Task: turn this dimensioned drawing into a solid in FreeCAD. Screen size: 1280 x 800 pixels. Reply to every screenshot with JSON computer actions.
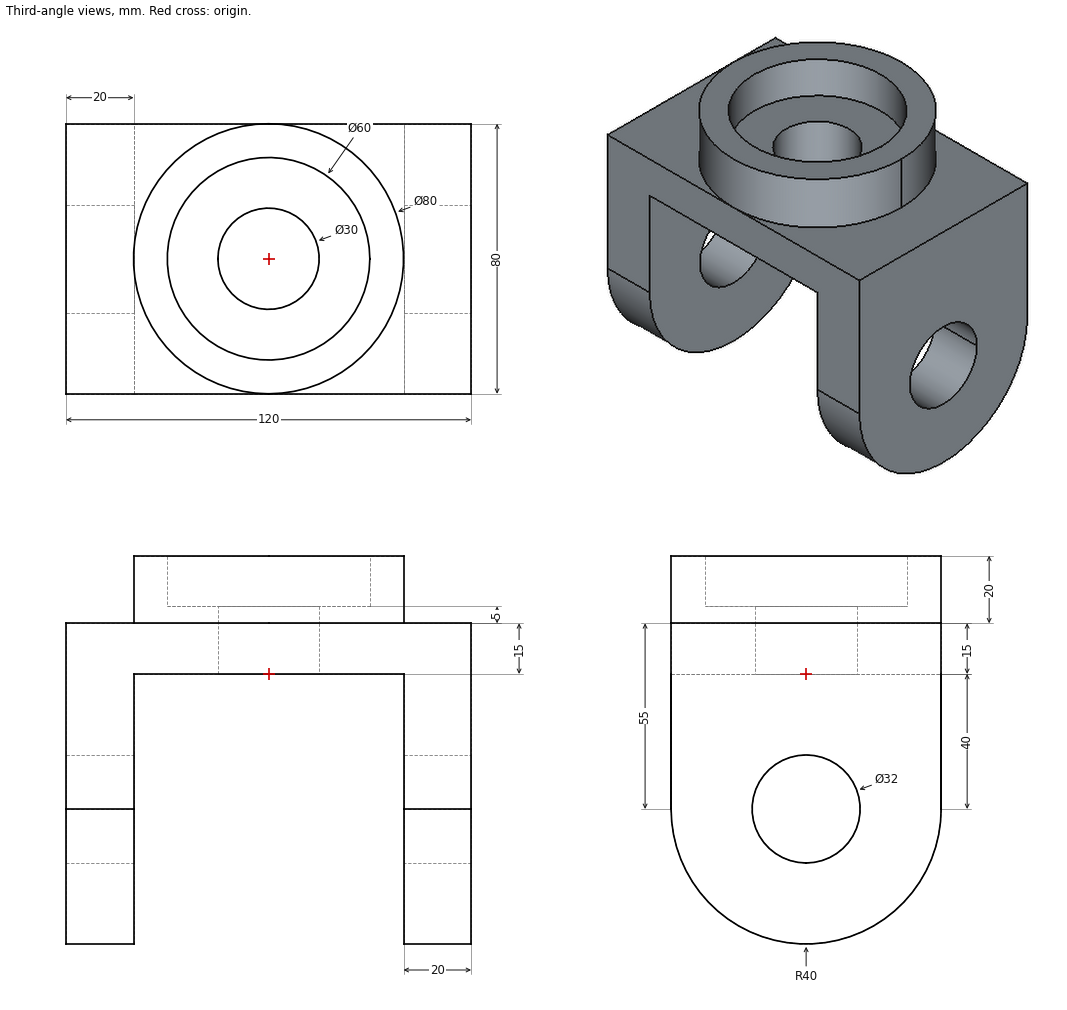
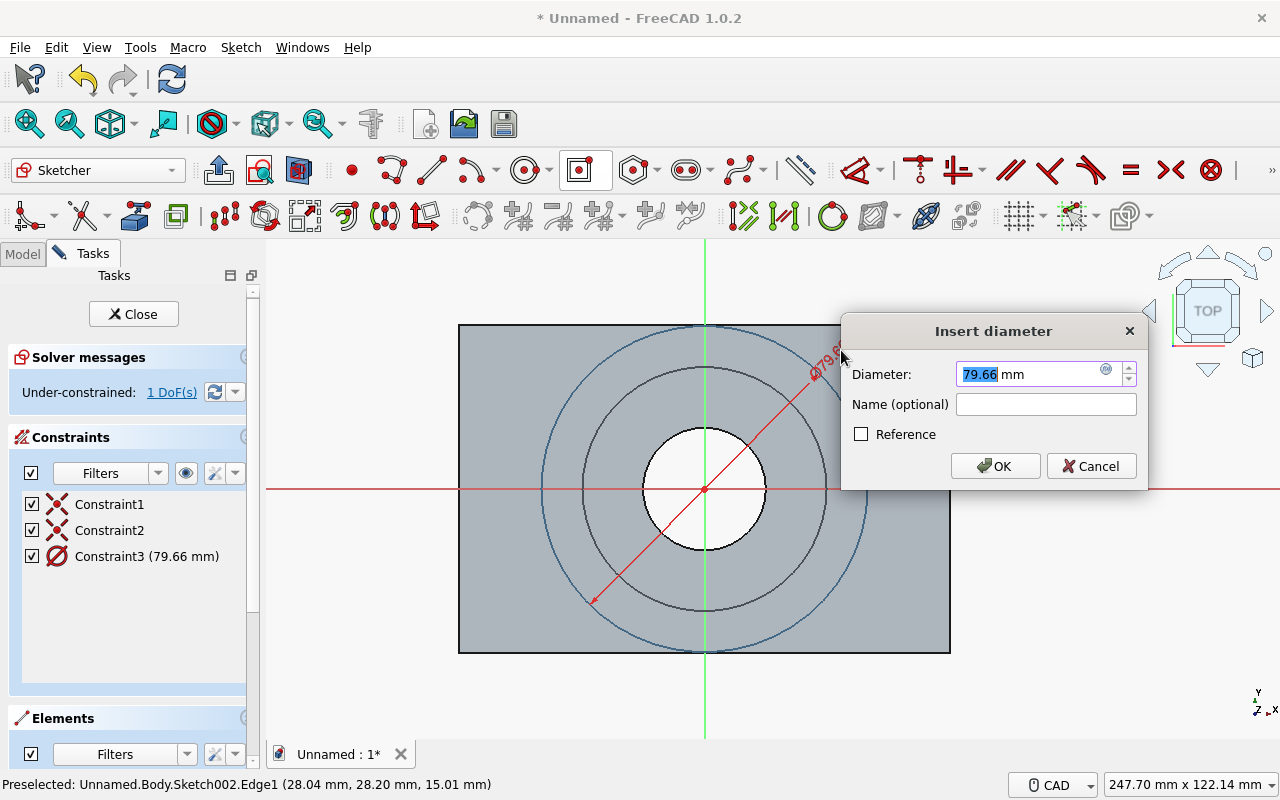
{"action": "type", "text": "80"}
{"action": "key", "text": "Return"}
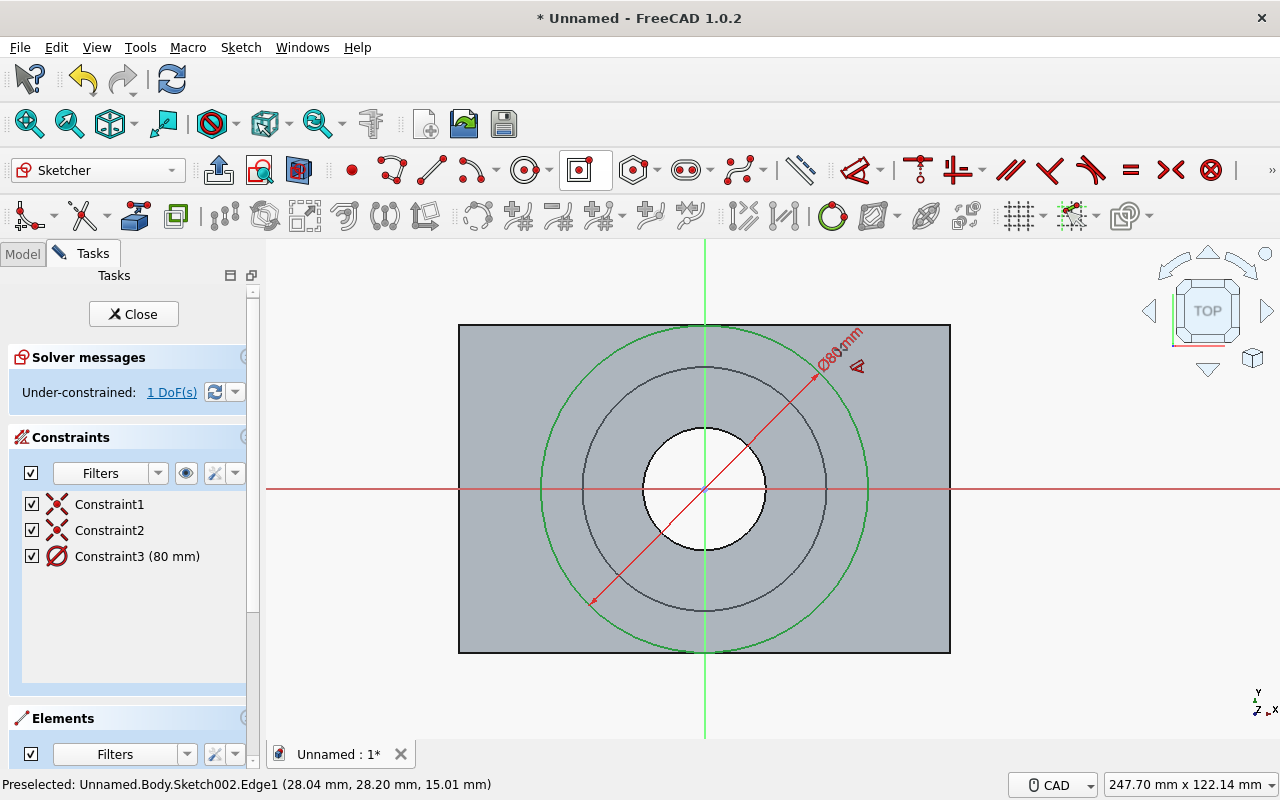
{"action": "left_click", "coordinate": [791, 403]}
{"action": "left_click", "coordinate": [874, 440]}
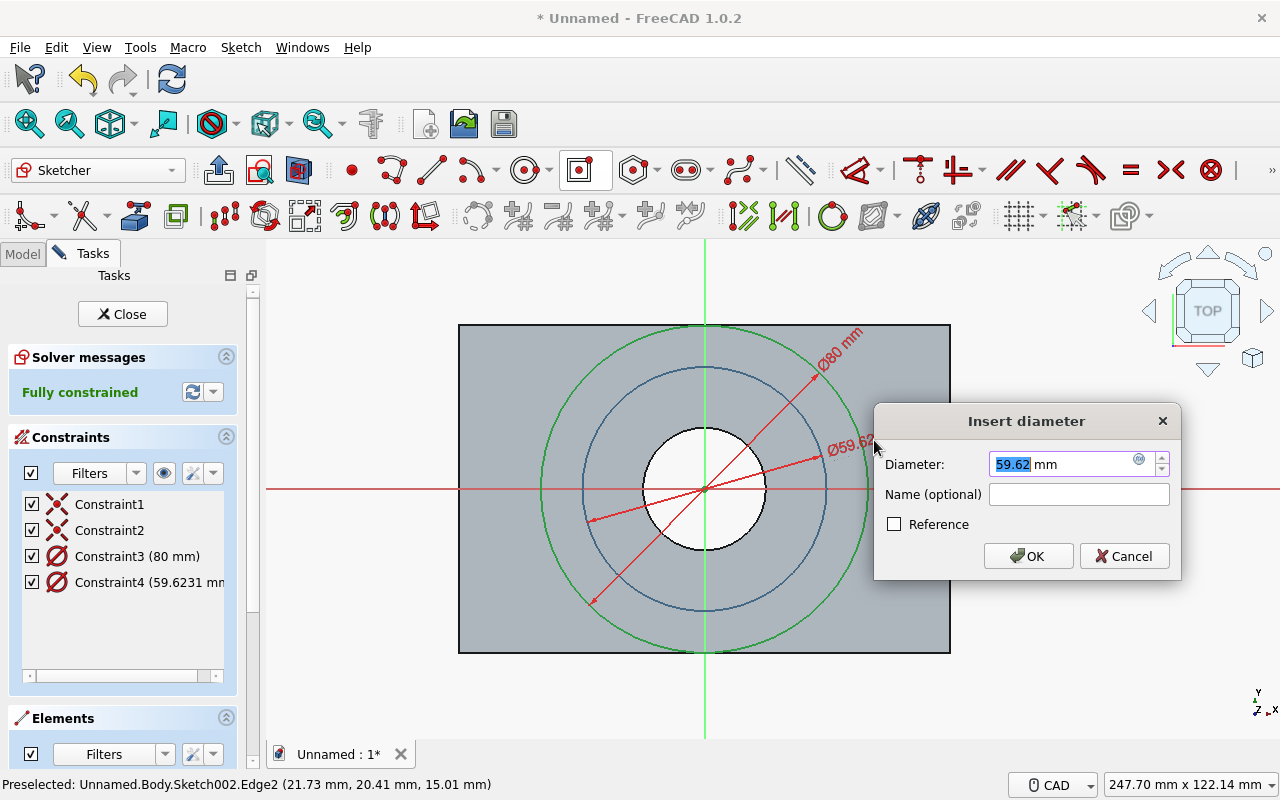
{"action": "type", "text": "60"}
{"action": "key", "text": "Return"}
{"action": "key", "text": "Escape"}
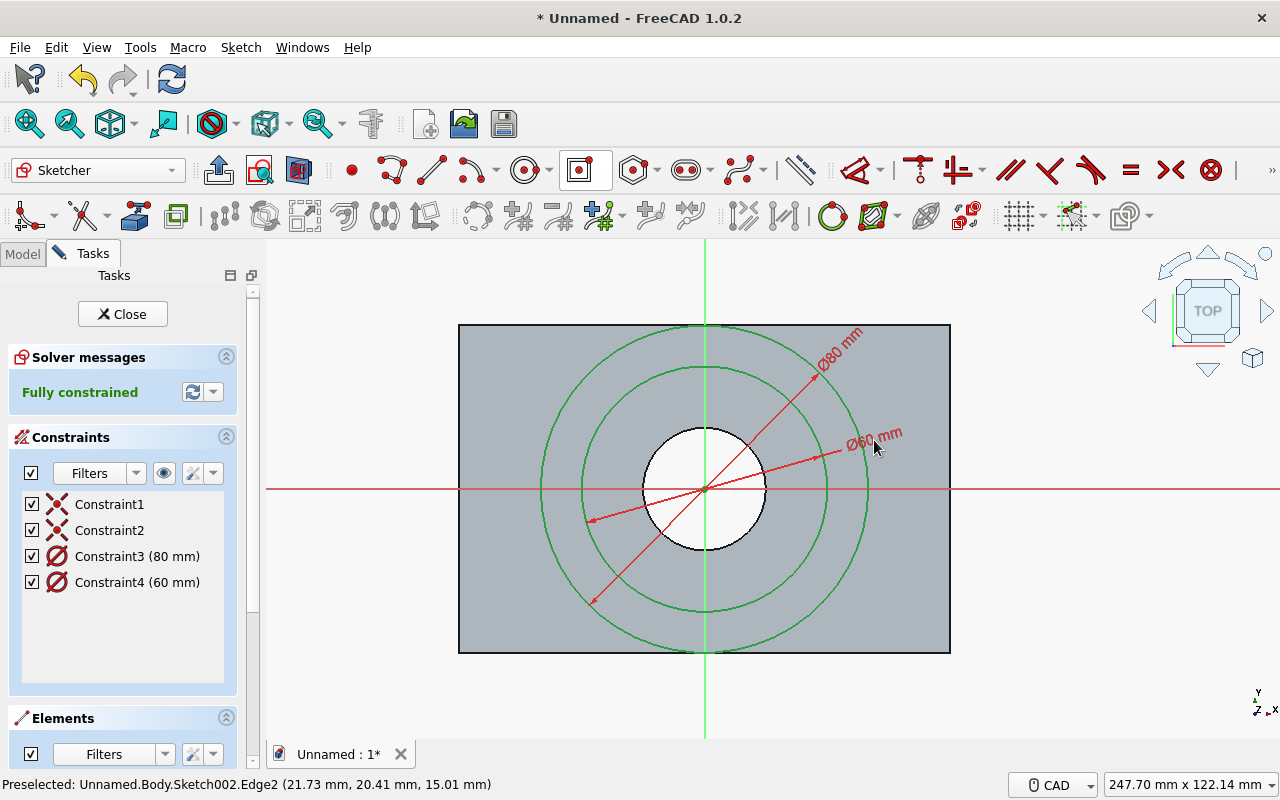
{"action": "left_click", "coordinate": [123, 314]}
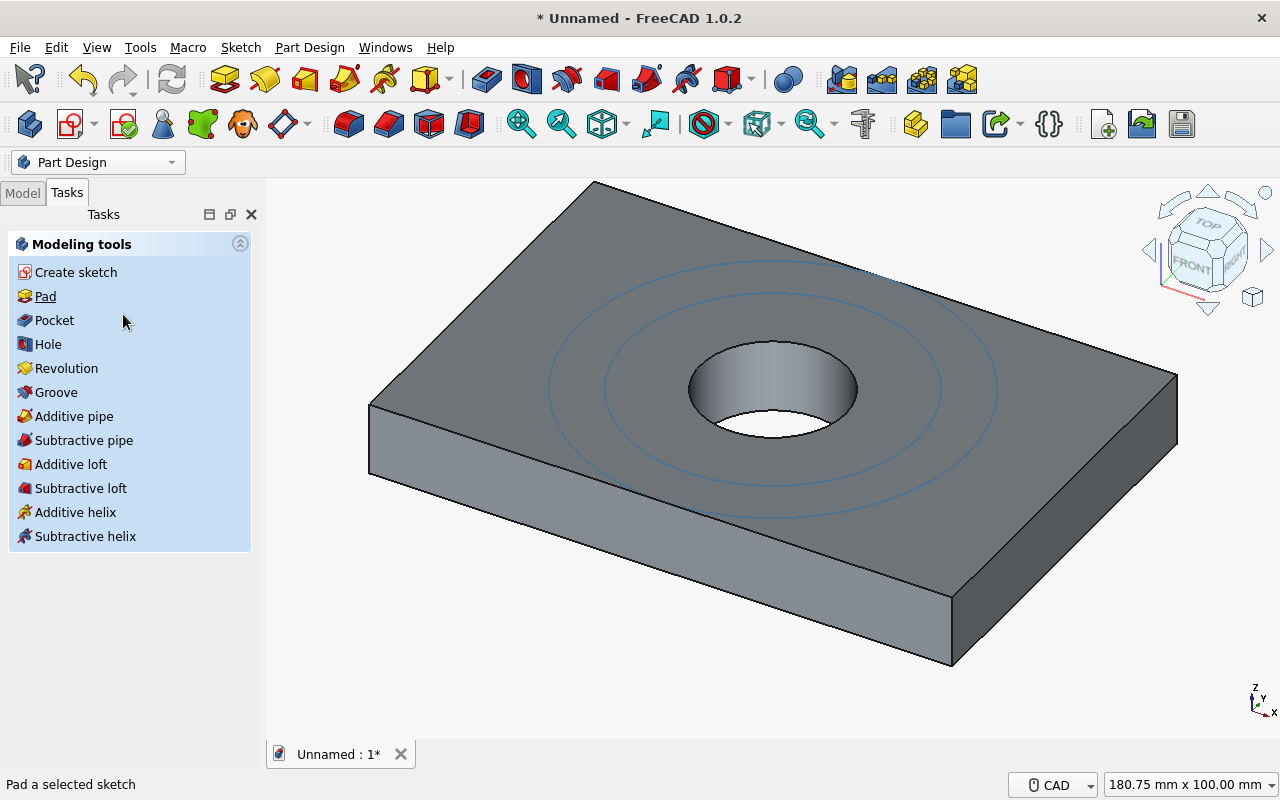
{"action": "left_click", "coordinate": [226, 80]}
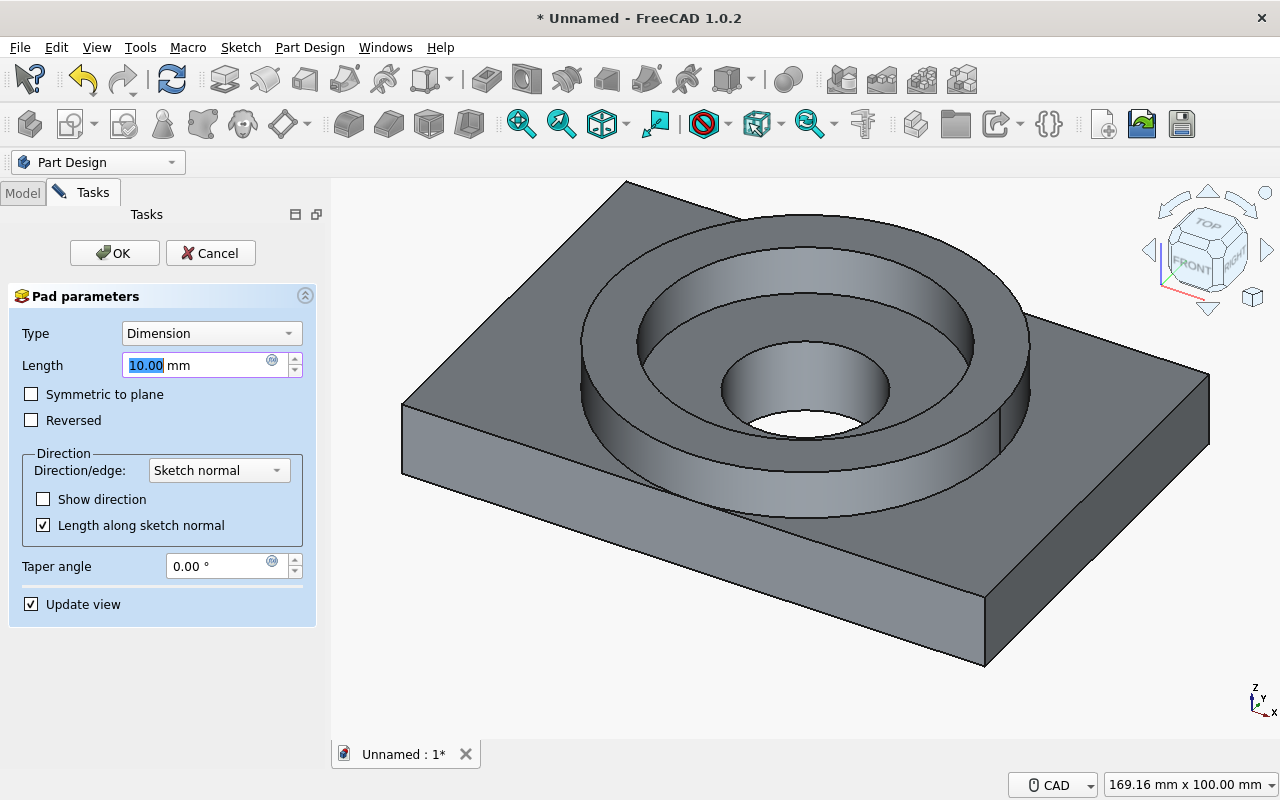
{"action": "type", "text": "20"}
{"action": "key", "text": "Tab"}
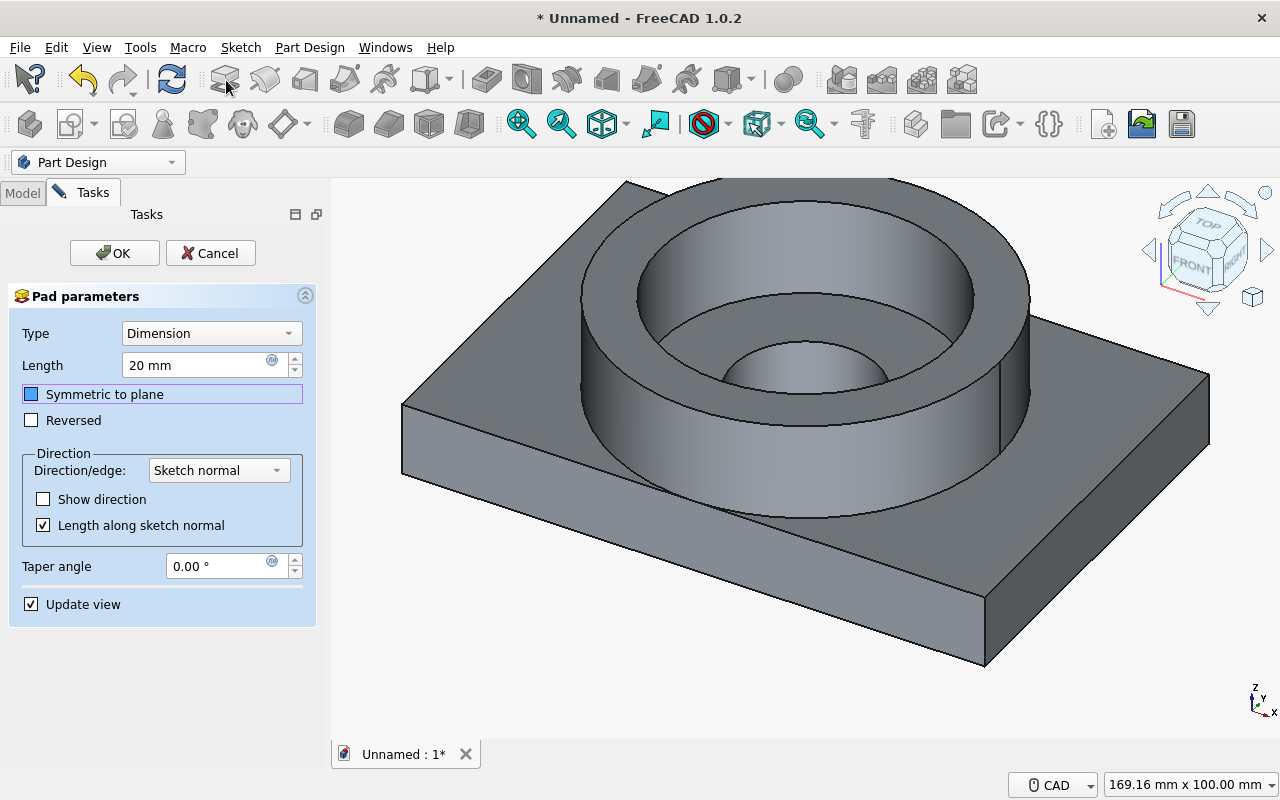
{"action": "left_click", "coordinate": [115, 253]}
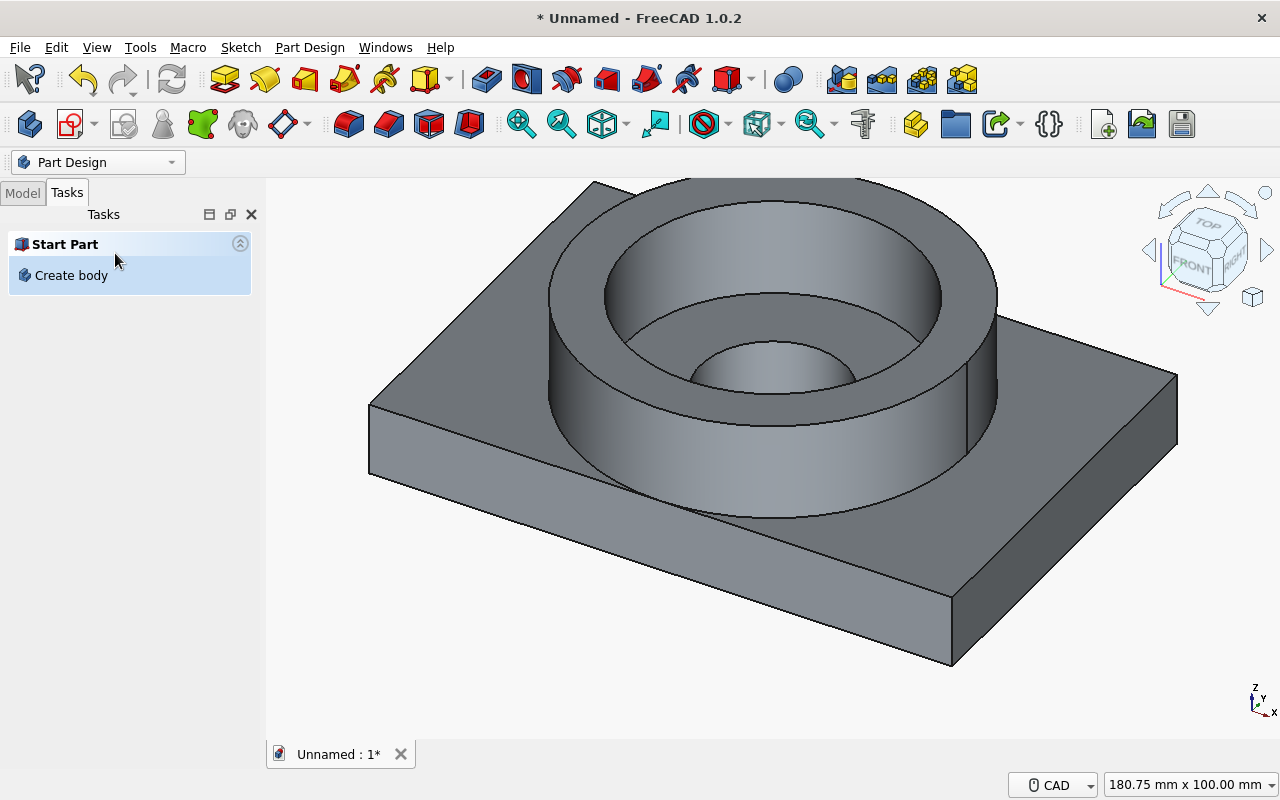
{"action": "left_click", "coordinate": [522, 124]}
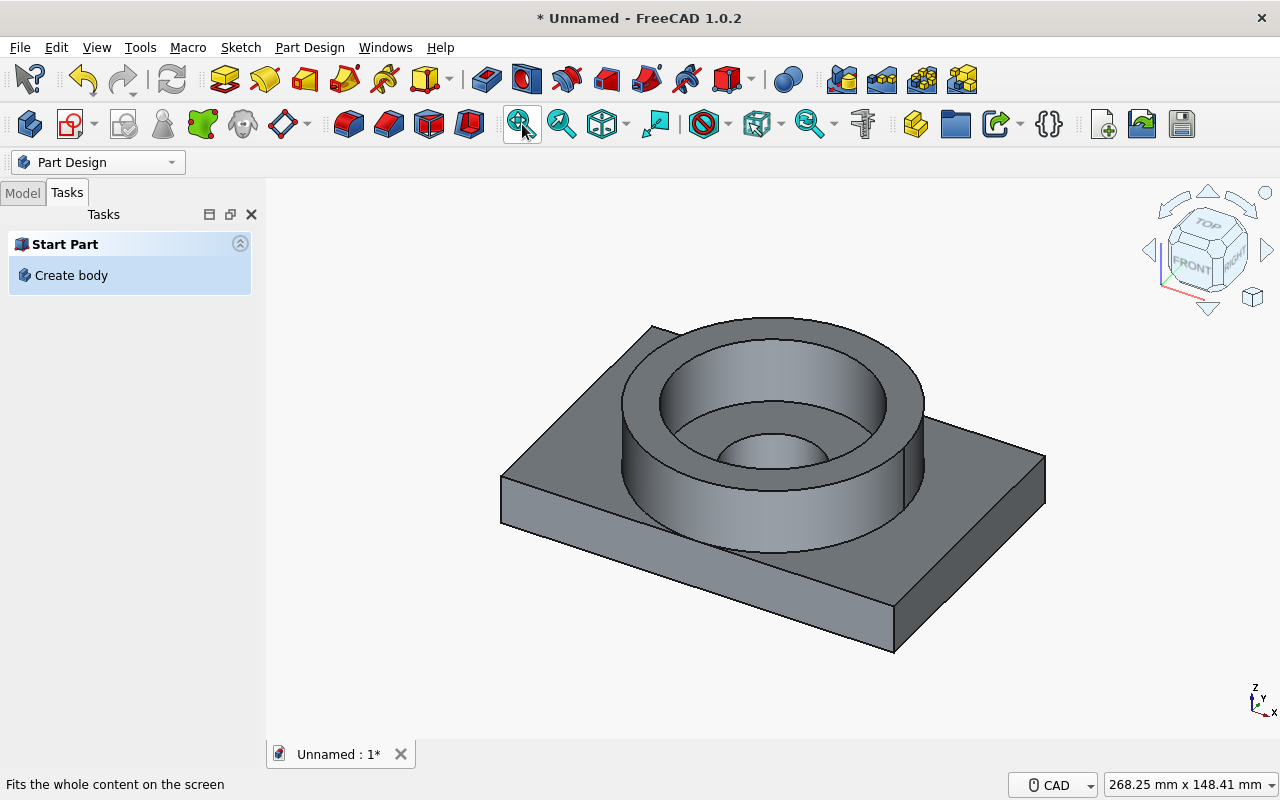
{"action": "left_click", "coordinate": [884, 559]}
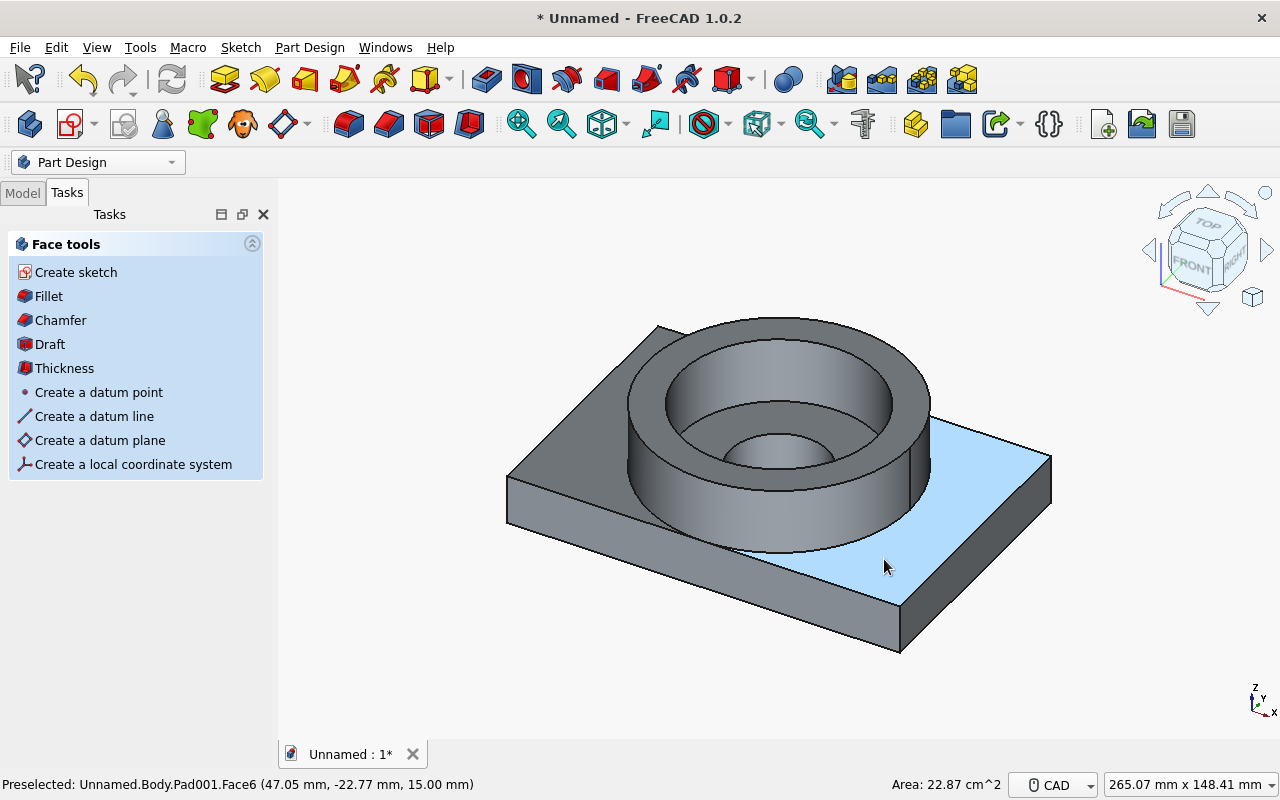
{"action": "left_click", "coordinate": [70, 124]}